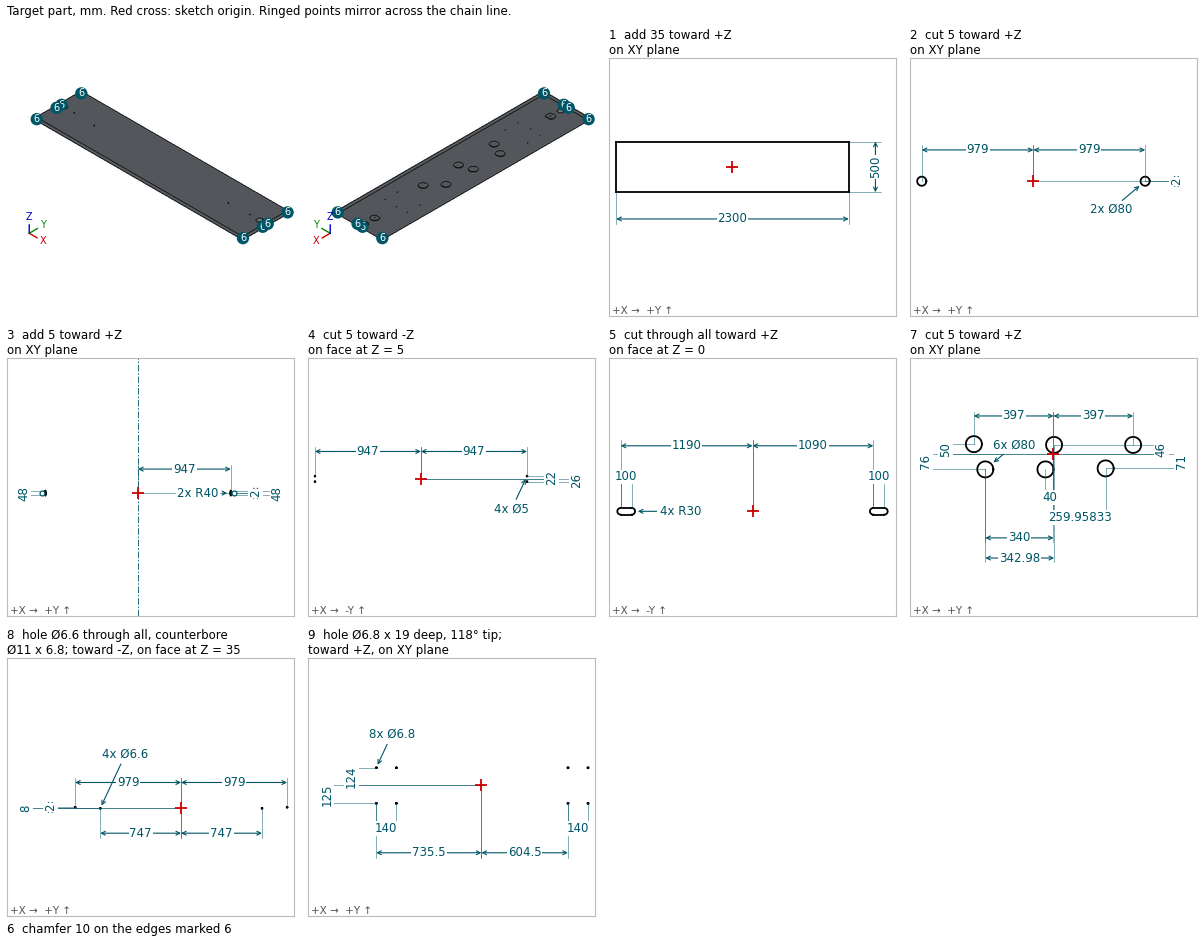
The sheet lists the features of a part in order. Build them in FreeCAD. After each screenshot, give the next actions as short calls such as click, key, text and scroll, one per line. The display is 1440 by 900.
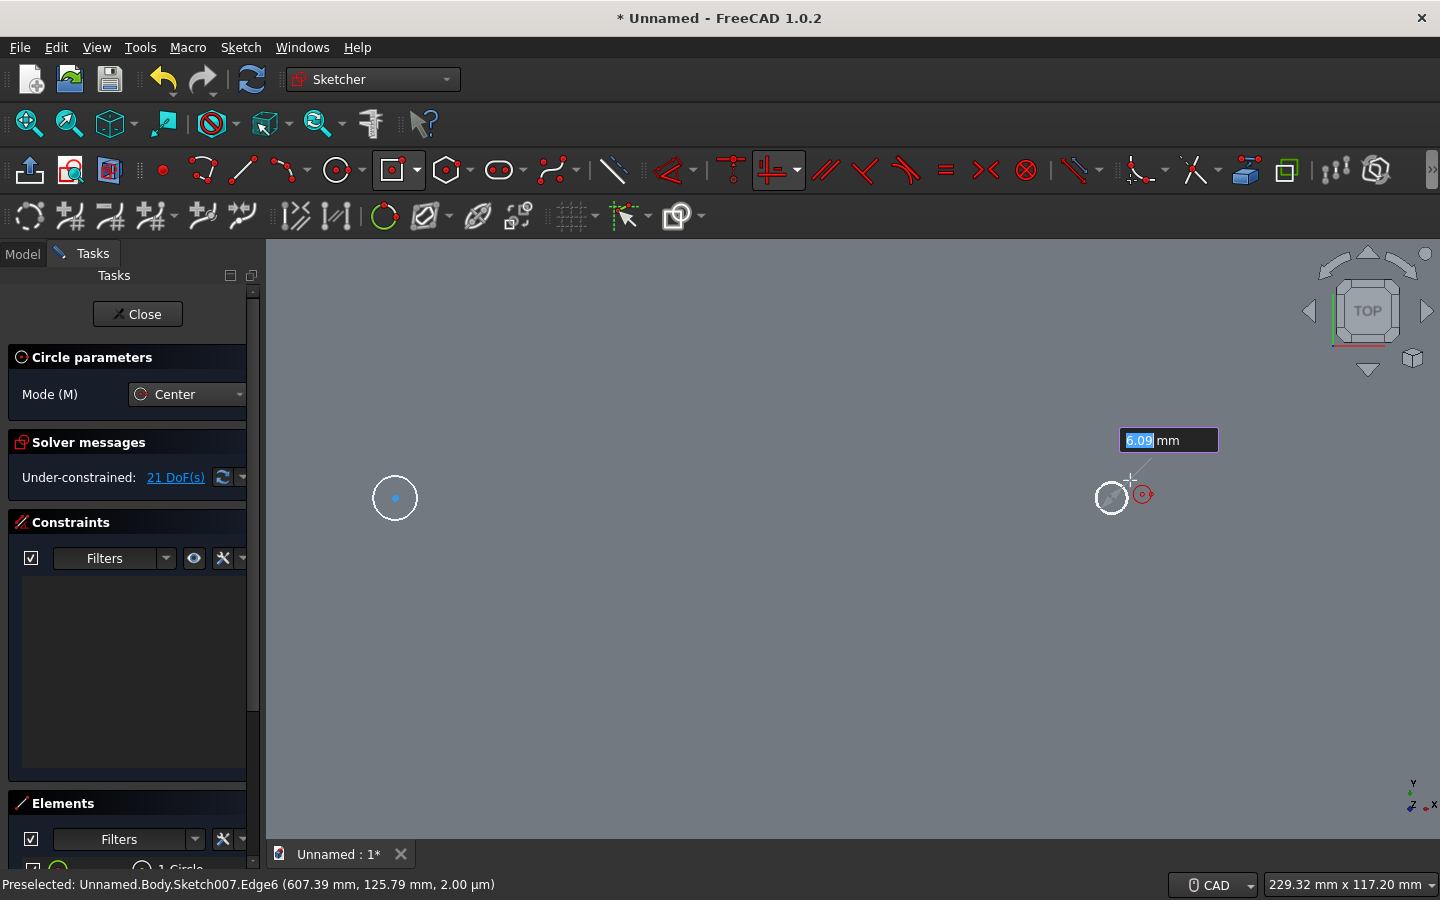
click(1121, 477)
key(Escape)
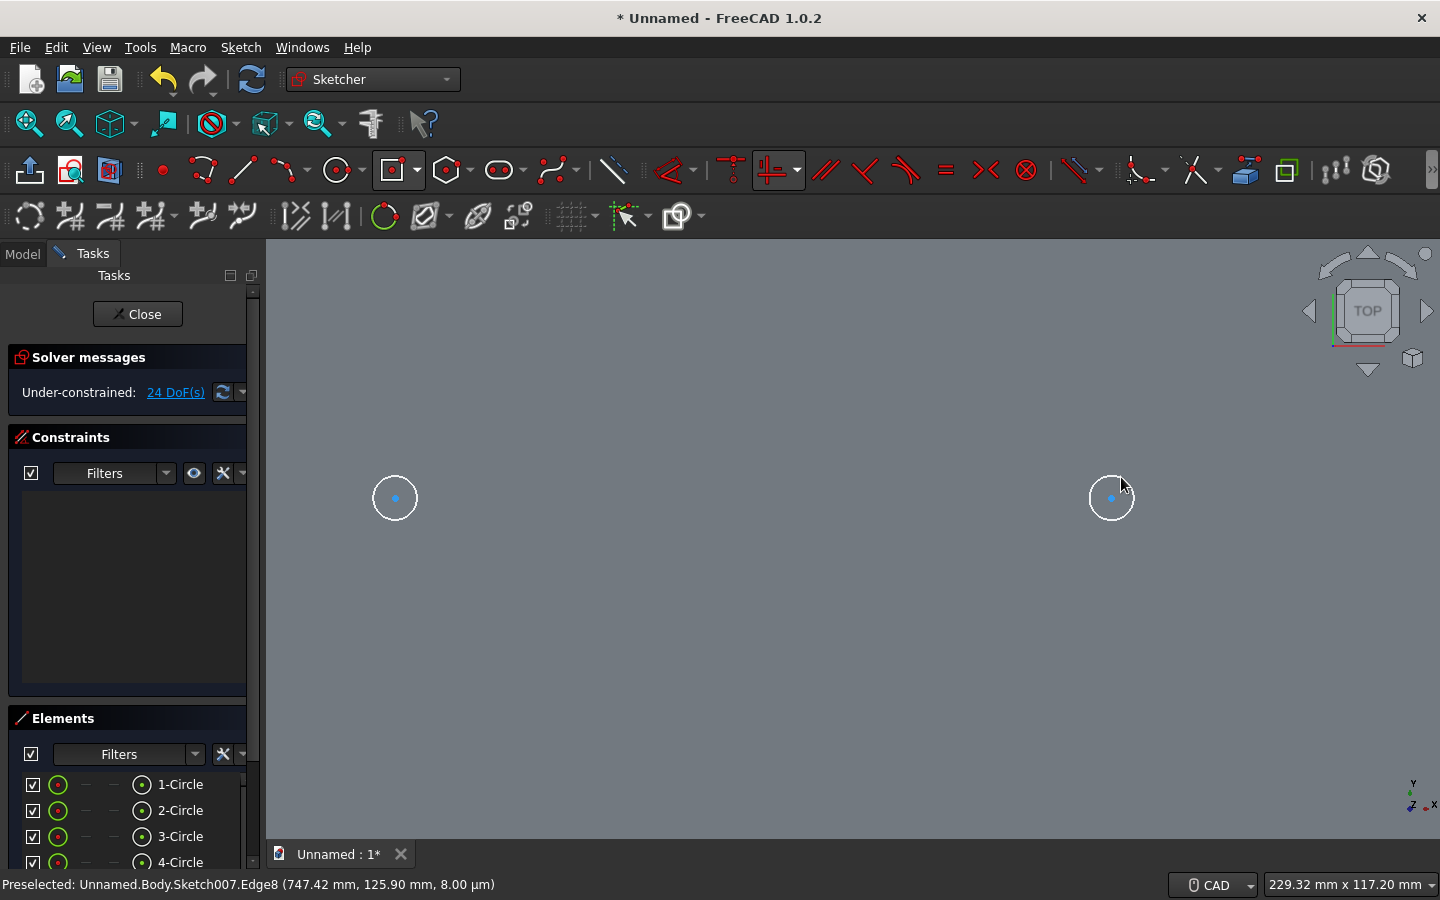
scroll(1130, 480, down, 12)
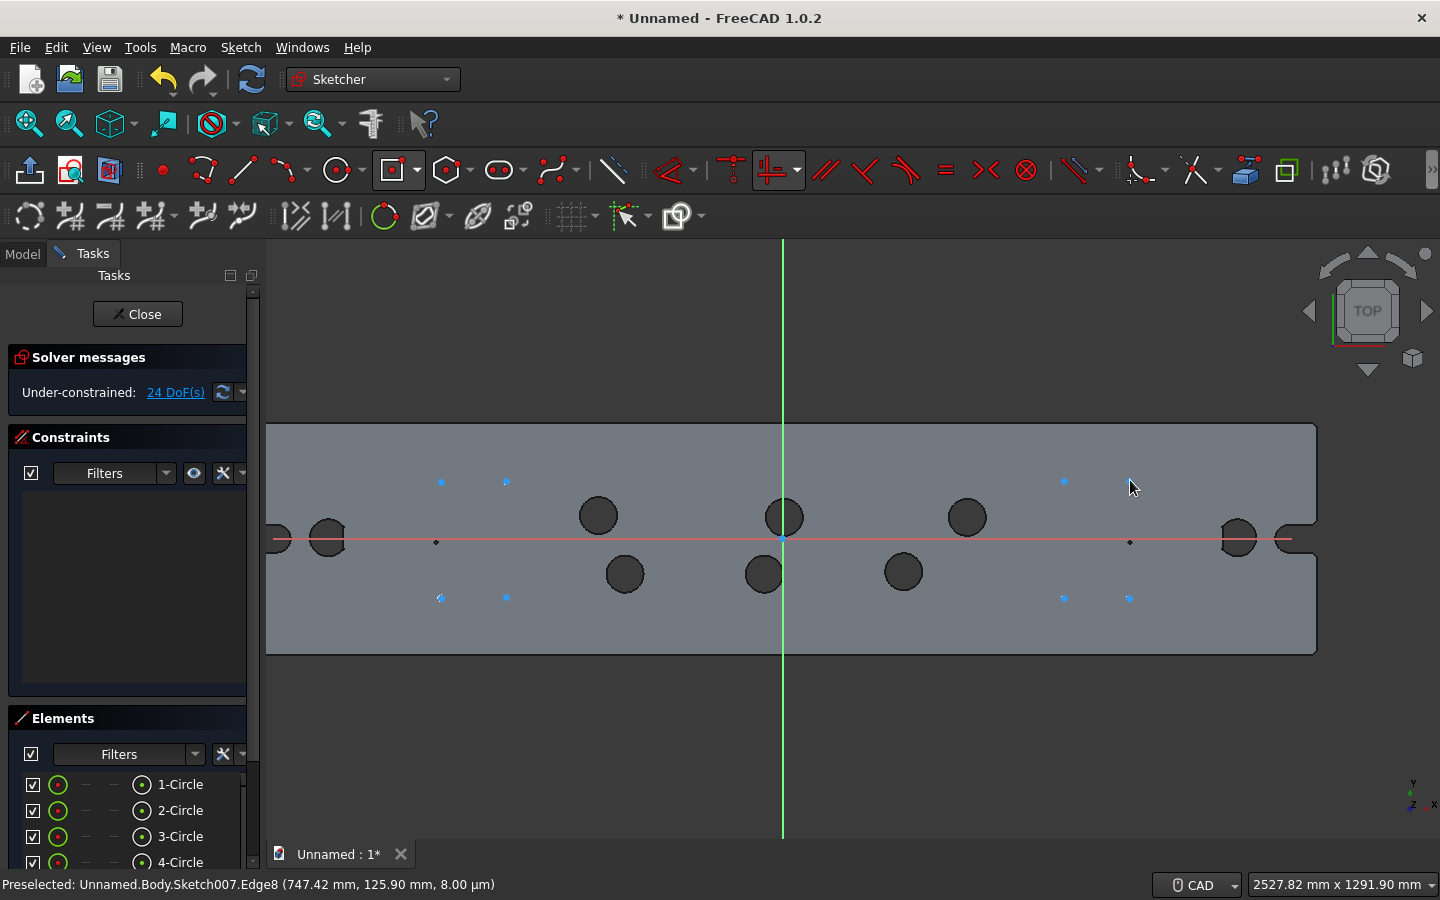
scroll(443, 596, up, 8)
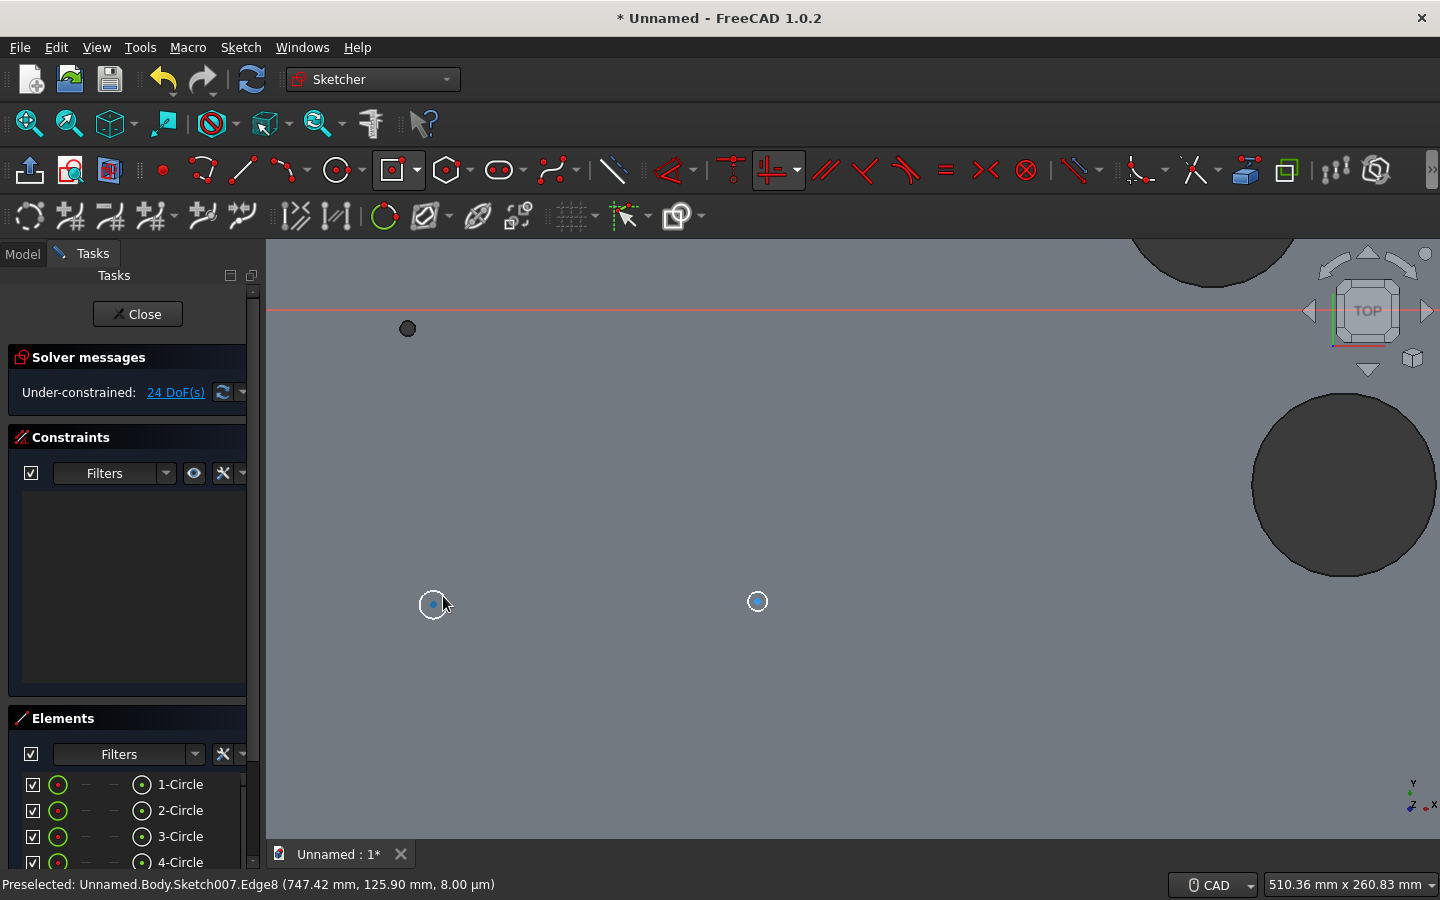
click(443, 595)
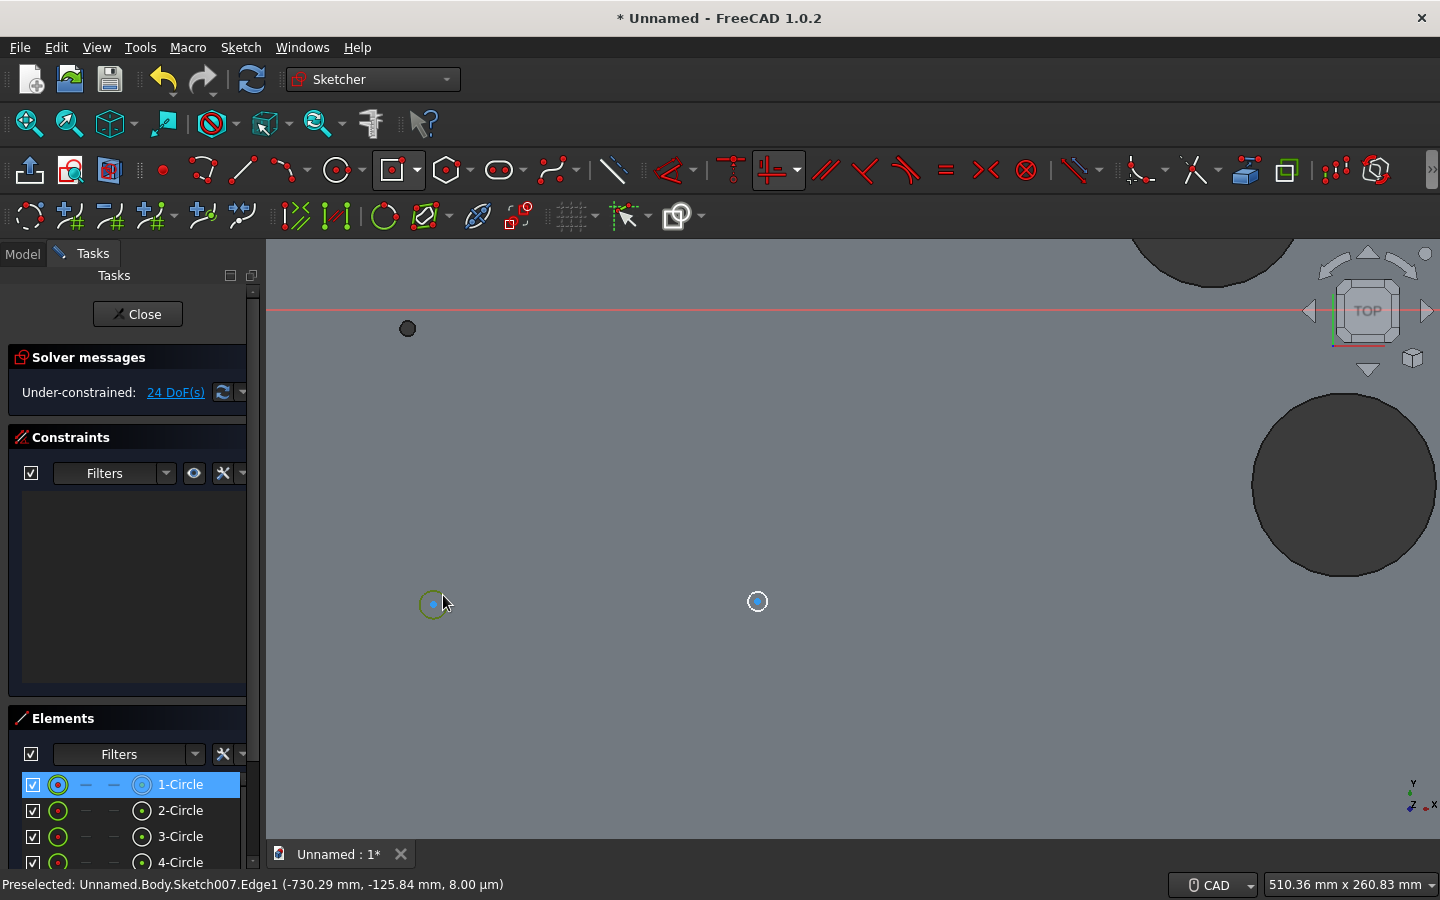
scroll(764, 595, up, 2)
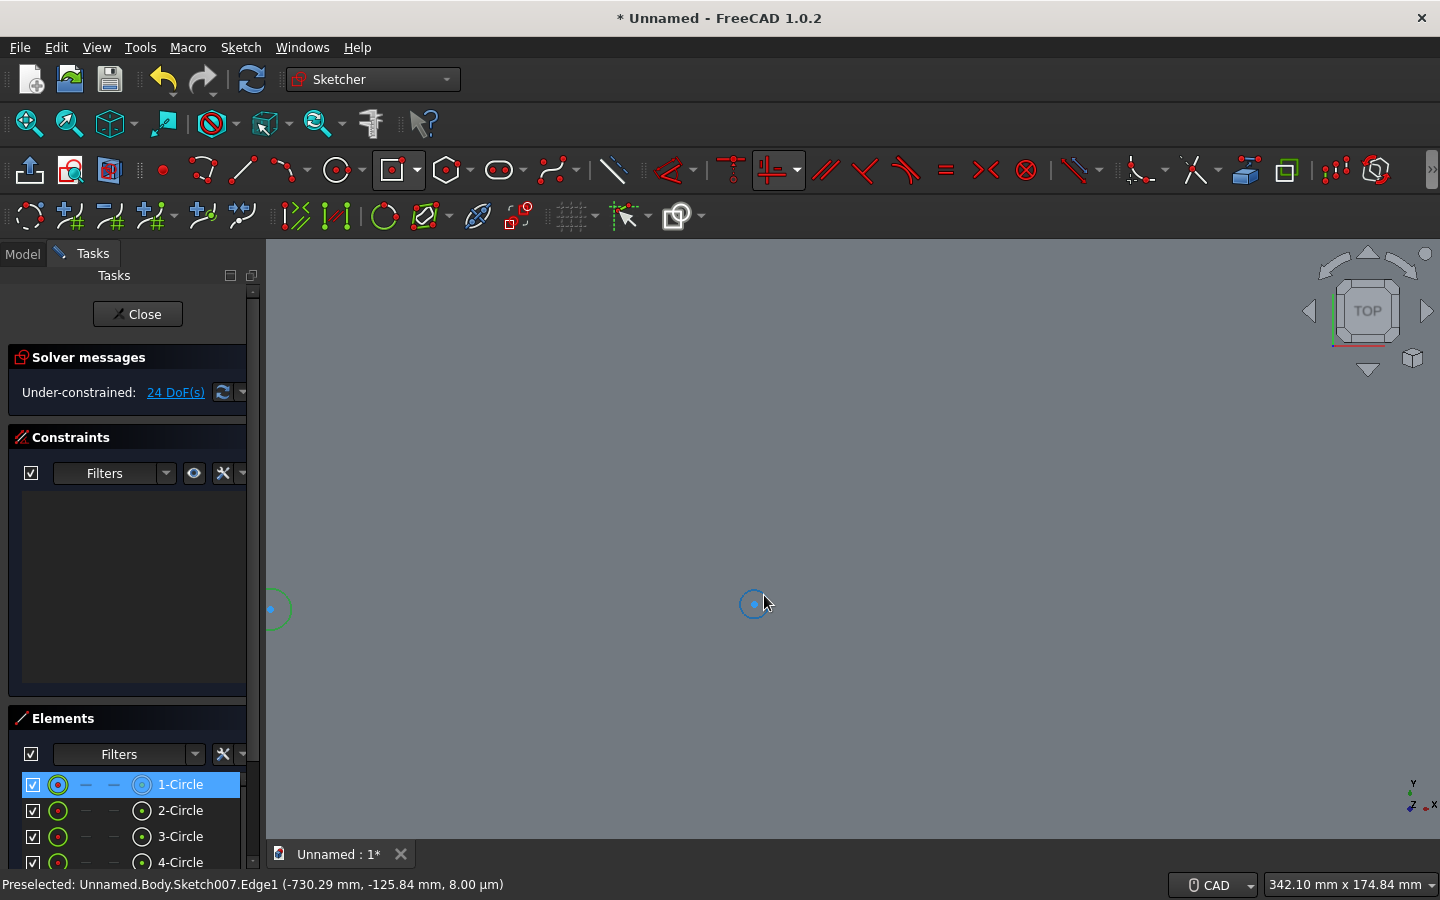
click(764, 594)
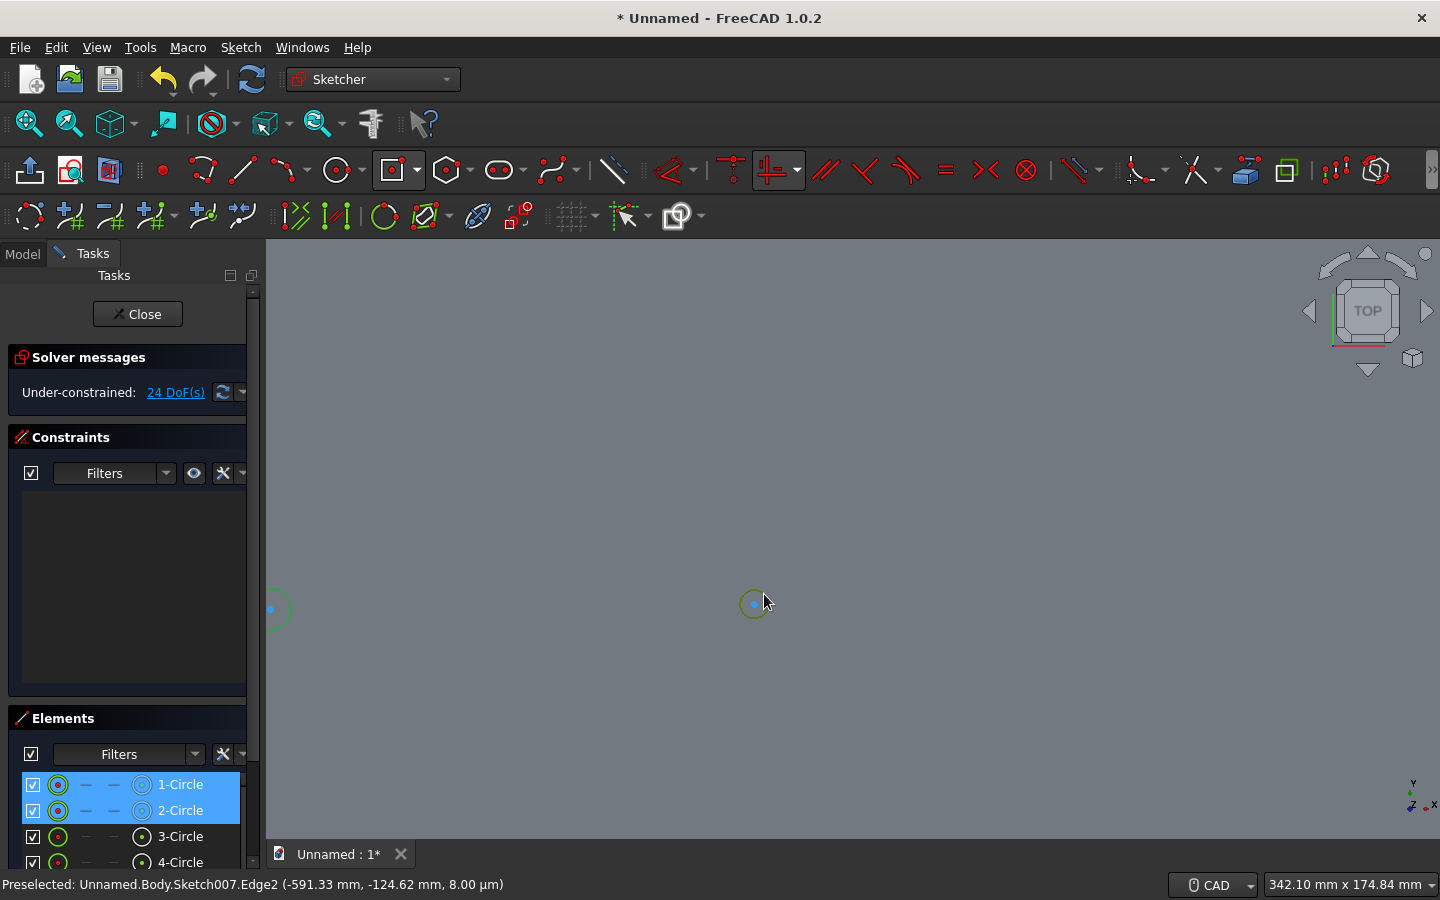
scroll(467, 597, down, 10)